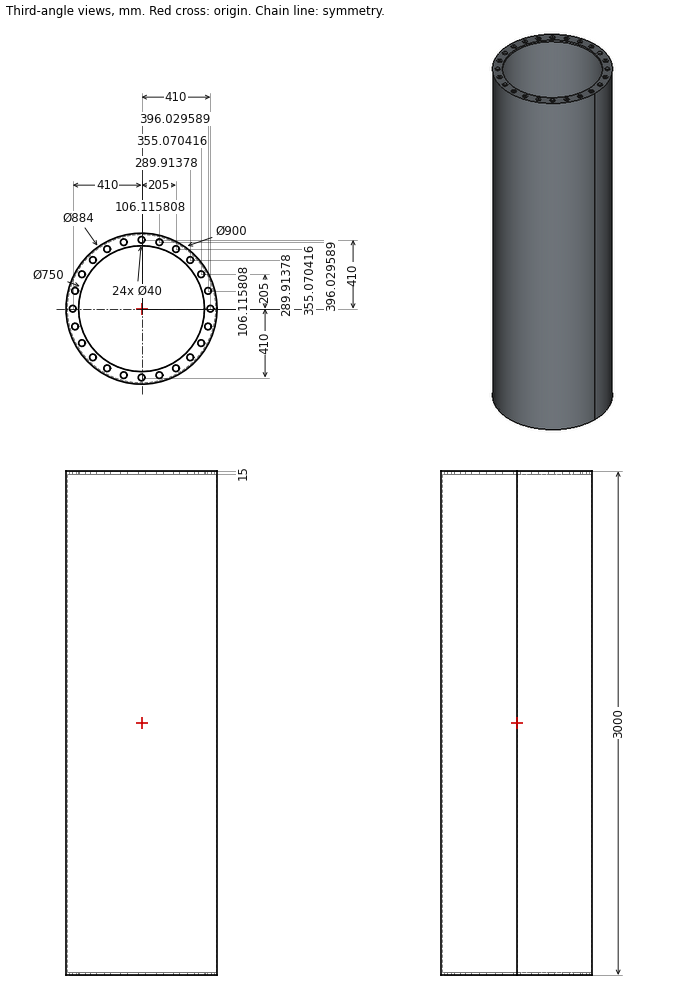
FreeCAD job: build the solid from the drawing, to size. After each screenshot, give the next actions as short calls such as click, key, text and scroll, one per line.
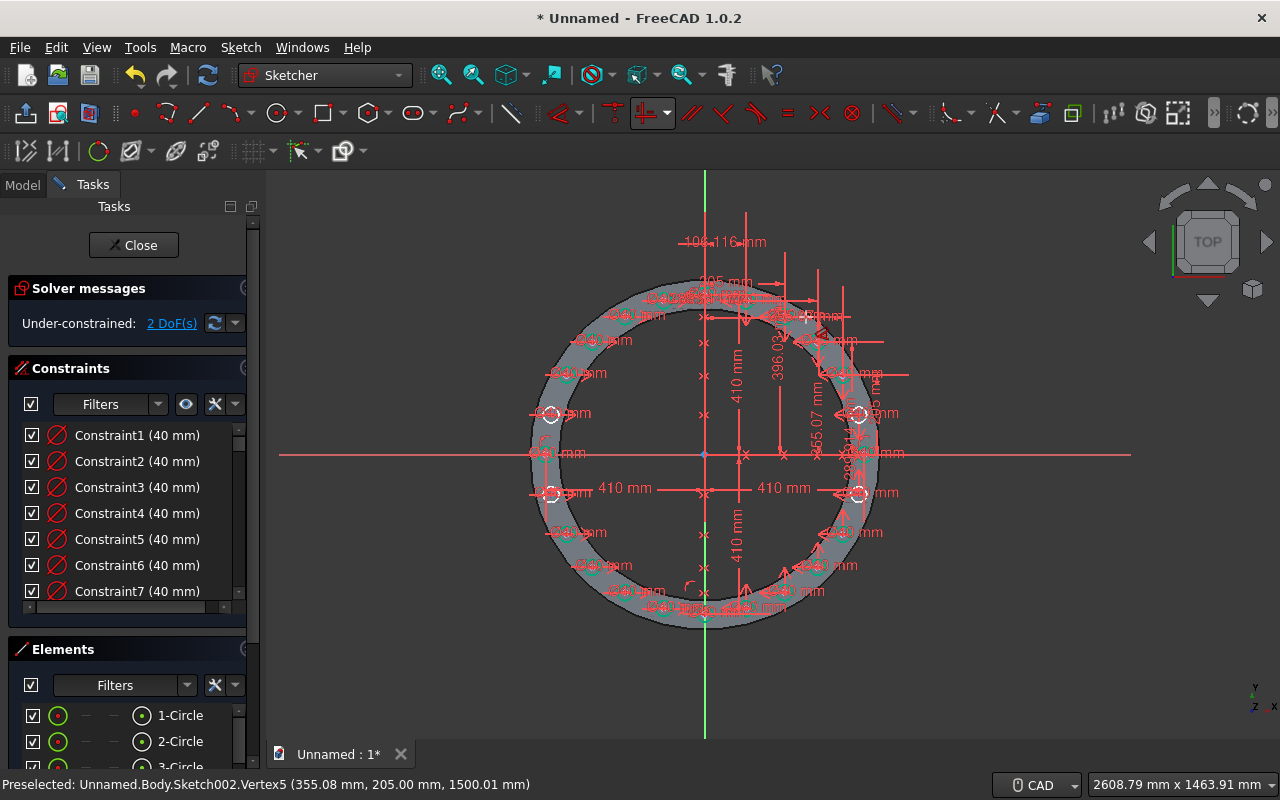
click(859, 415)
click(782, 513)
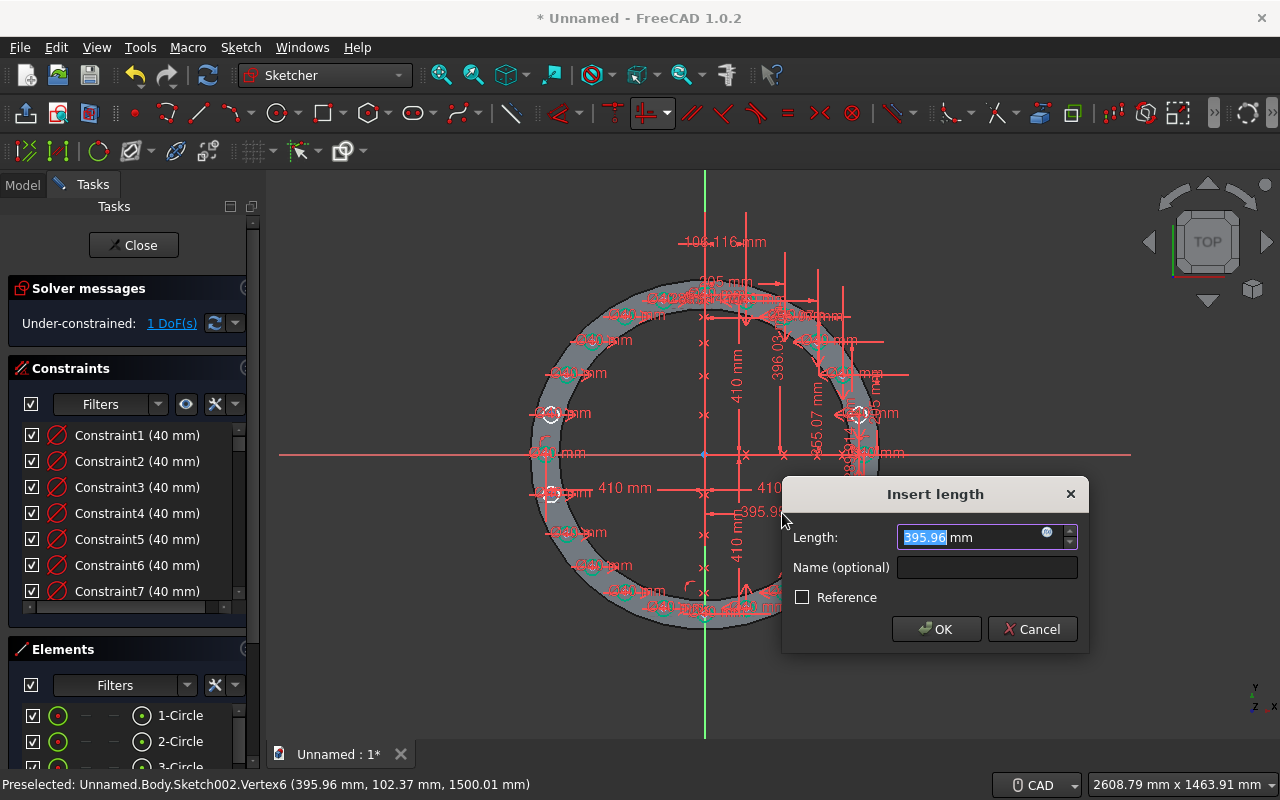
text(396.029589)
key(Return)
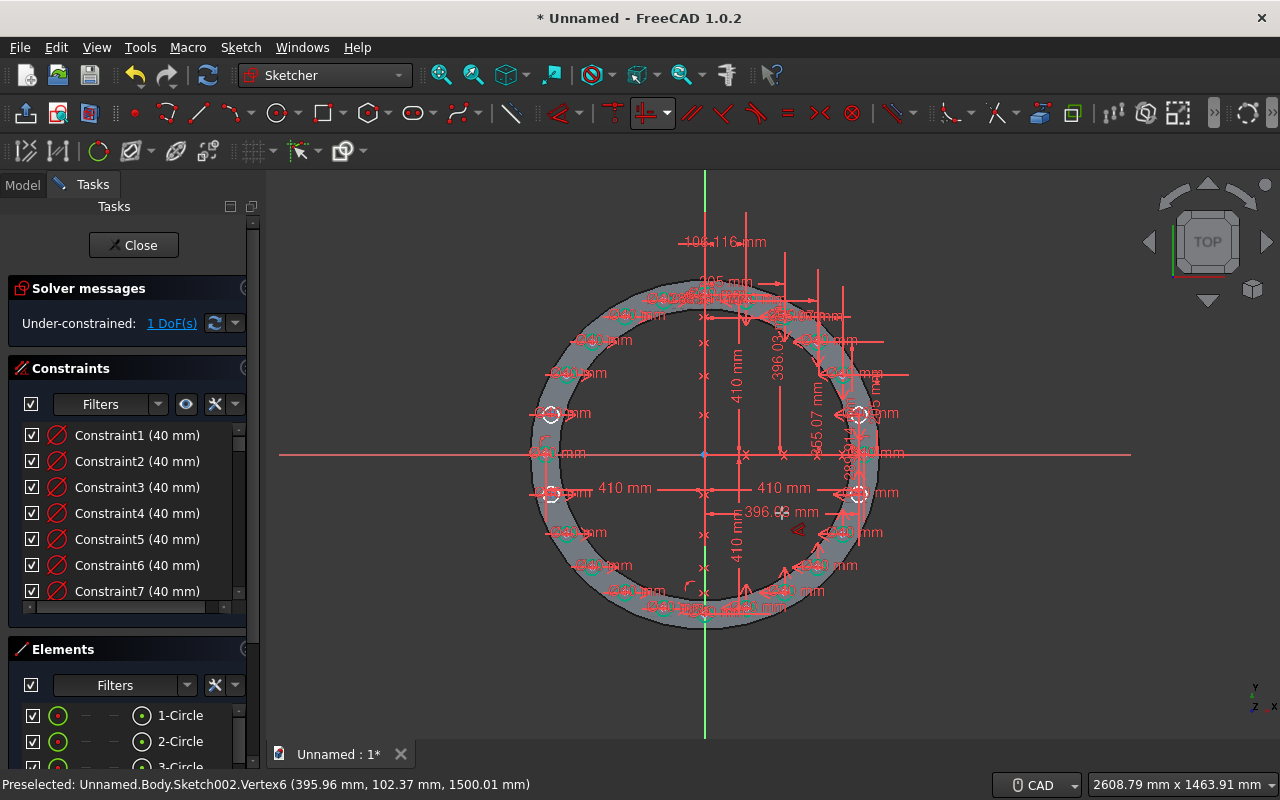
click(859, 415)
click(671, 435)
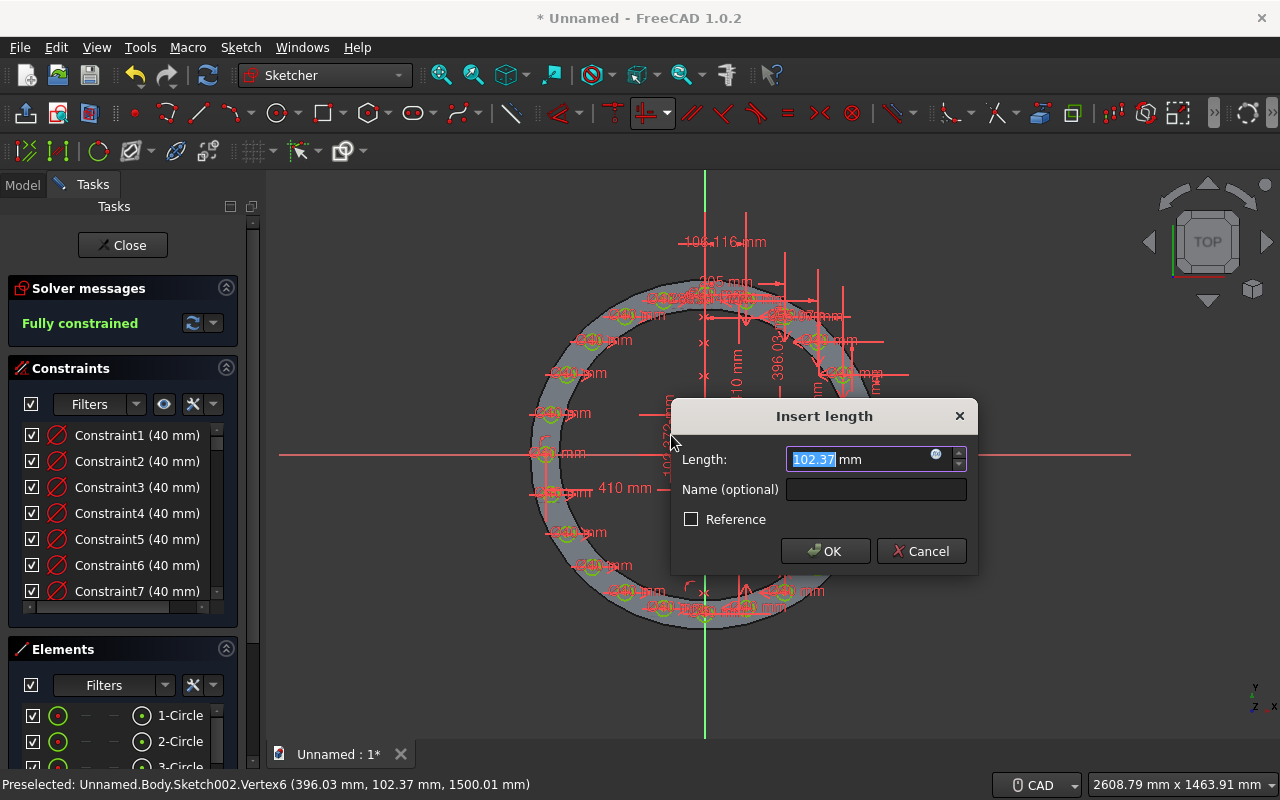
text(106.115808)
key(Return)
key(Escape)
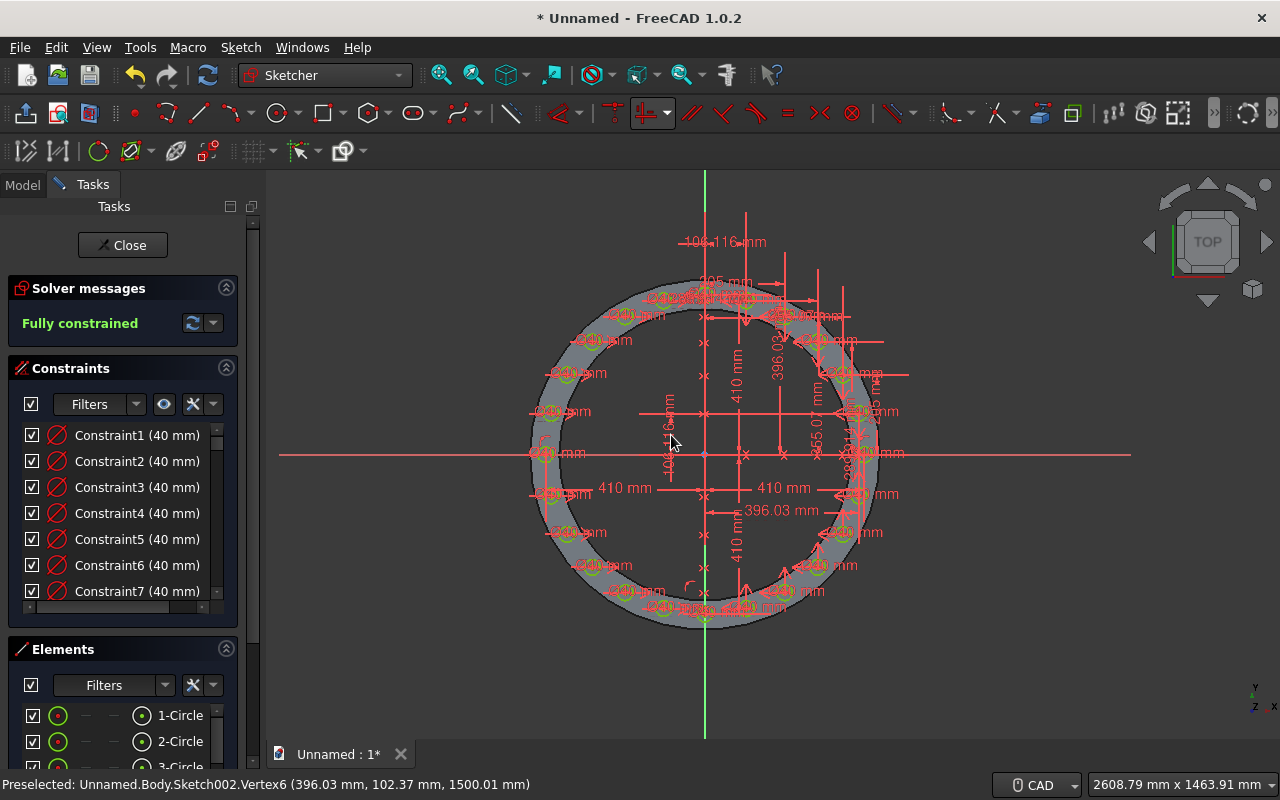
click(123, 245)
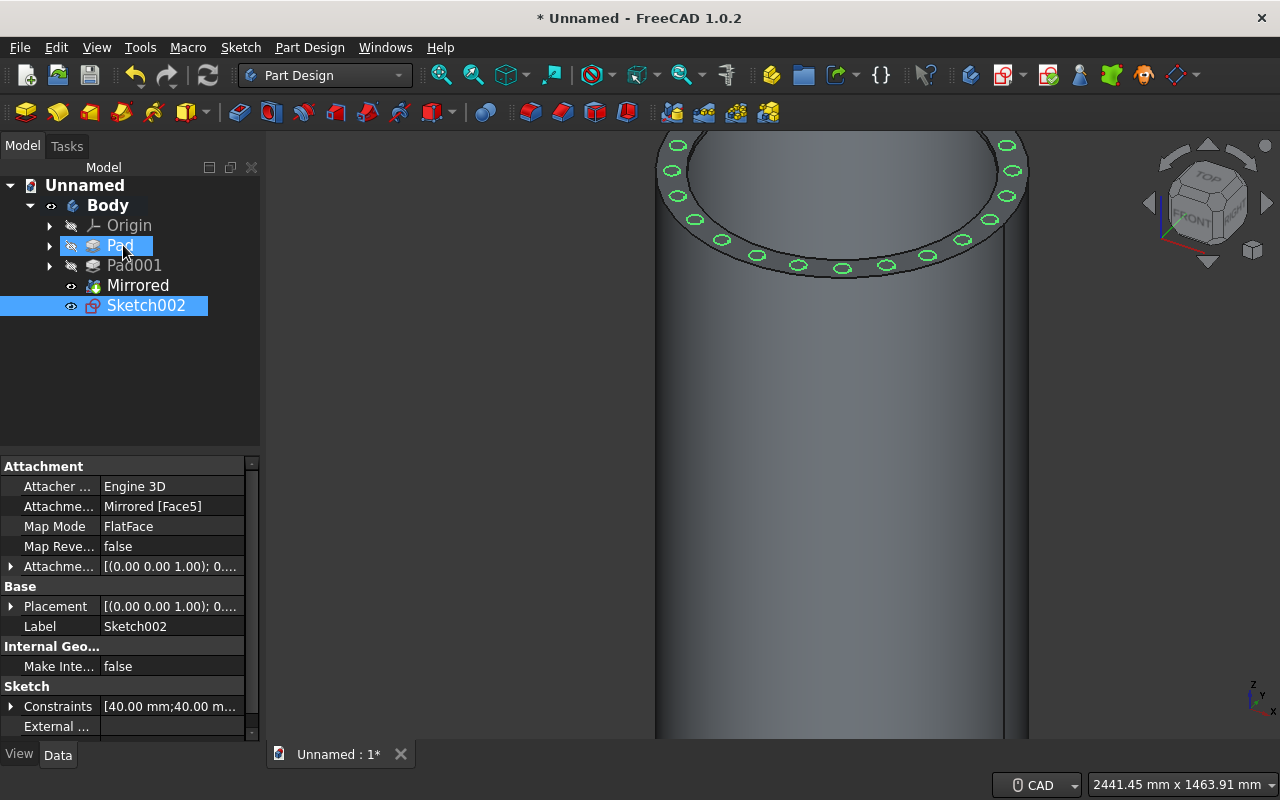
click(240, 112)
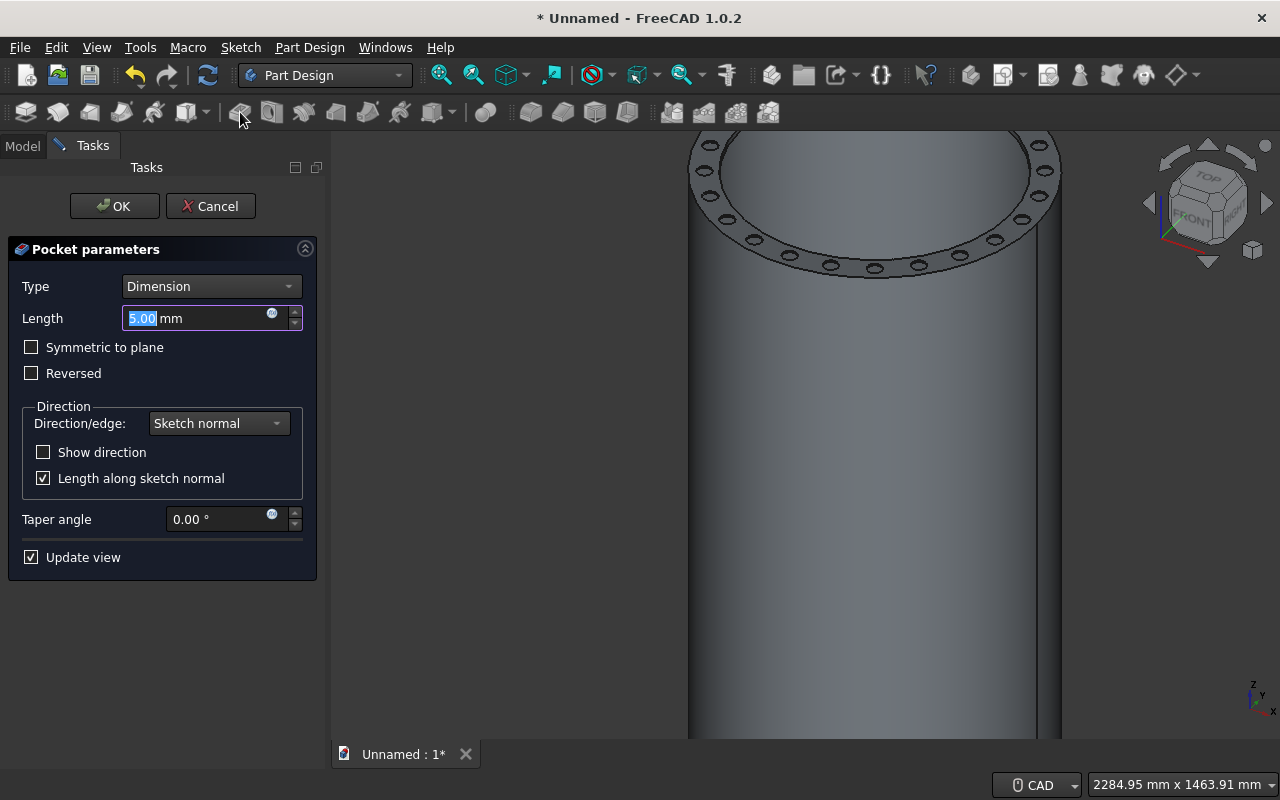
click(212, 286)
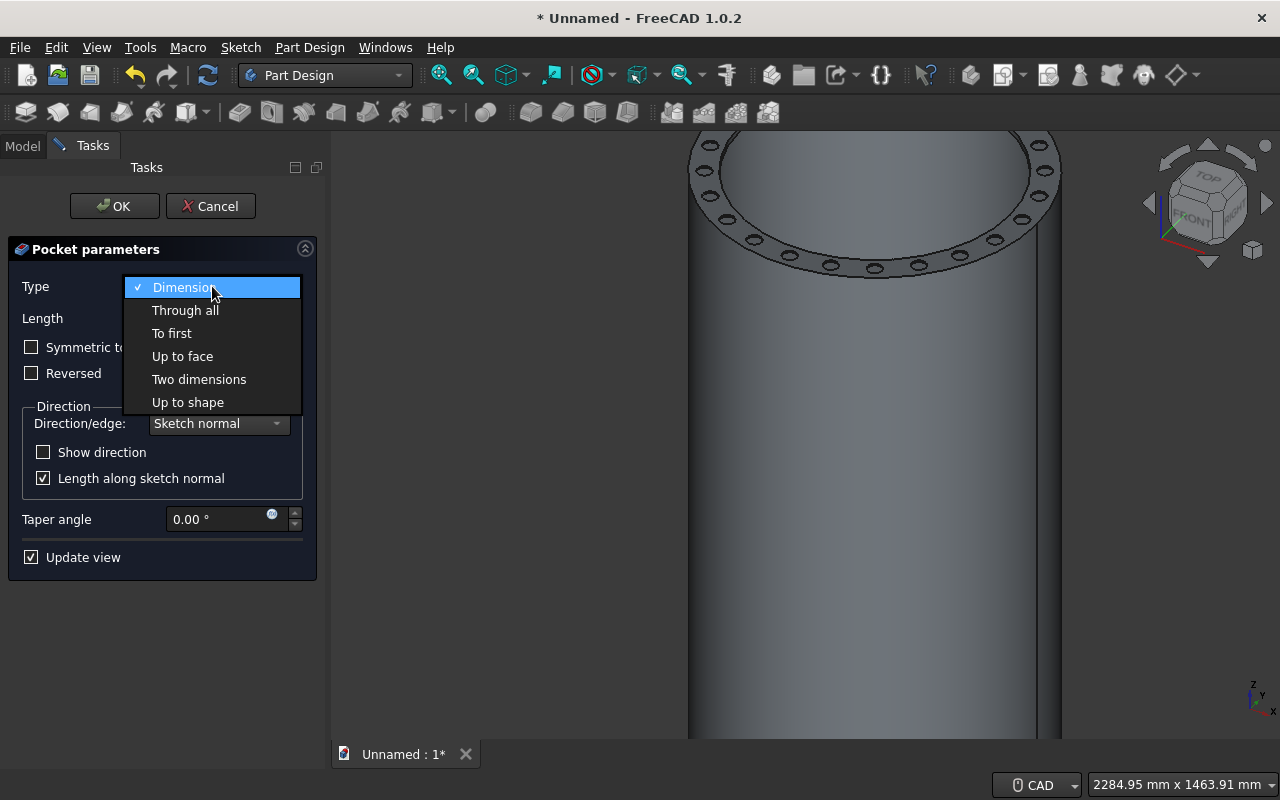
click(212, 310)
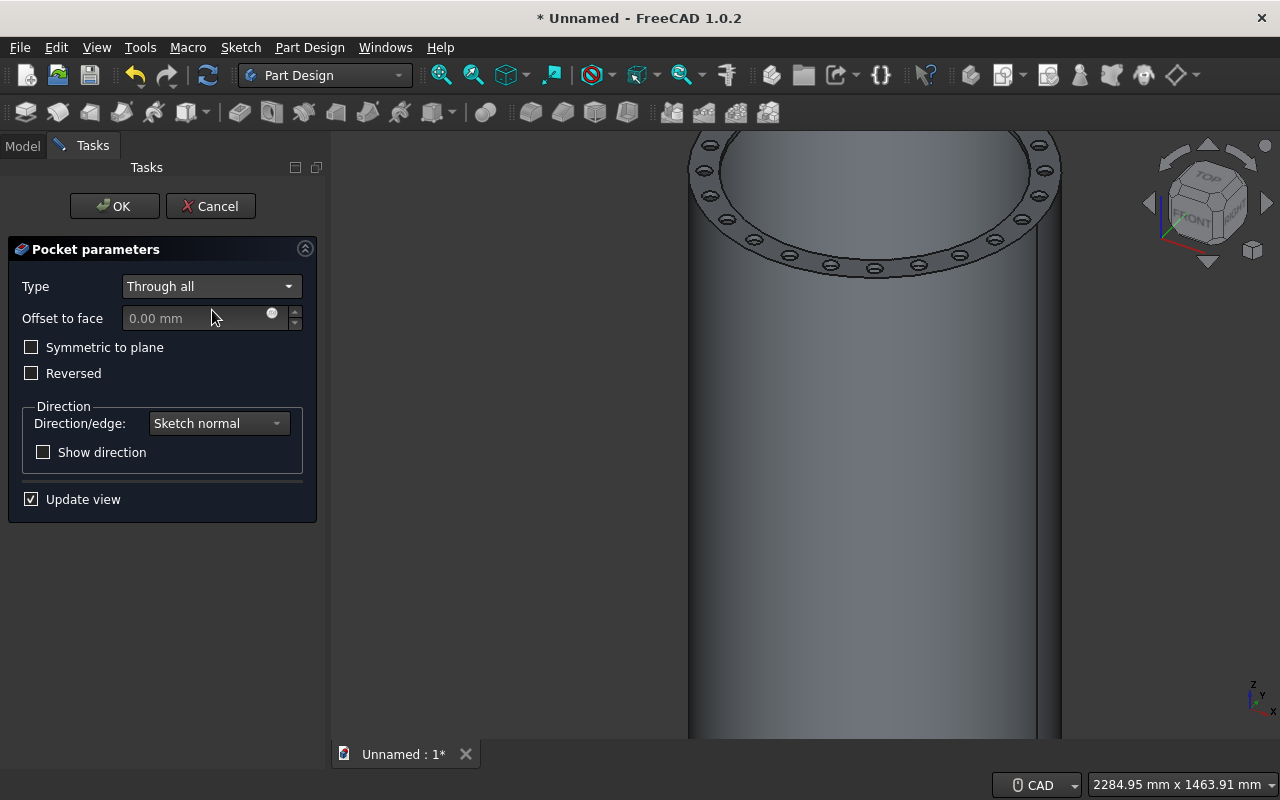
click(115, 206)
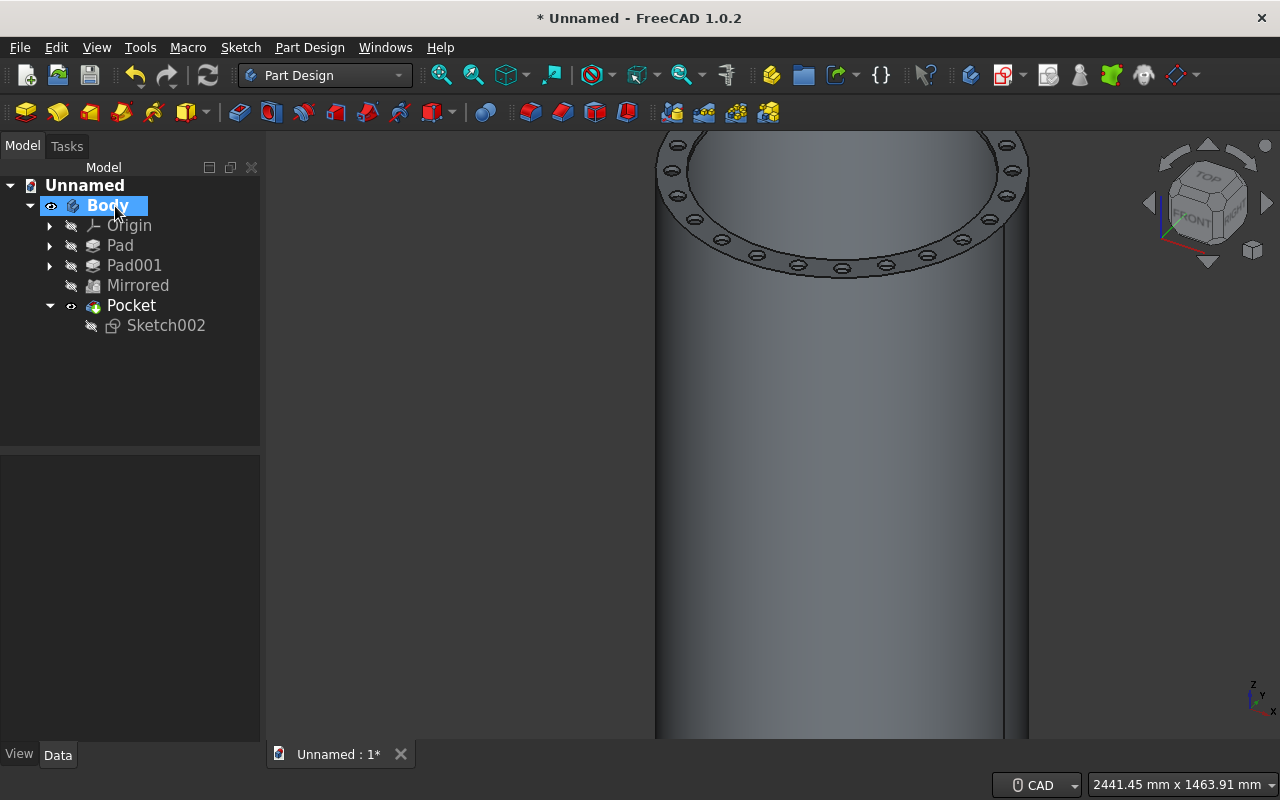
key(0)